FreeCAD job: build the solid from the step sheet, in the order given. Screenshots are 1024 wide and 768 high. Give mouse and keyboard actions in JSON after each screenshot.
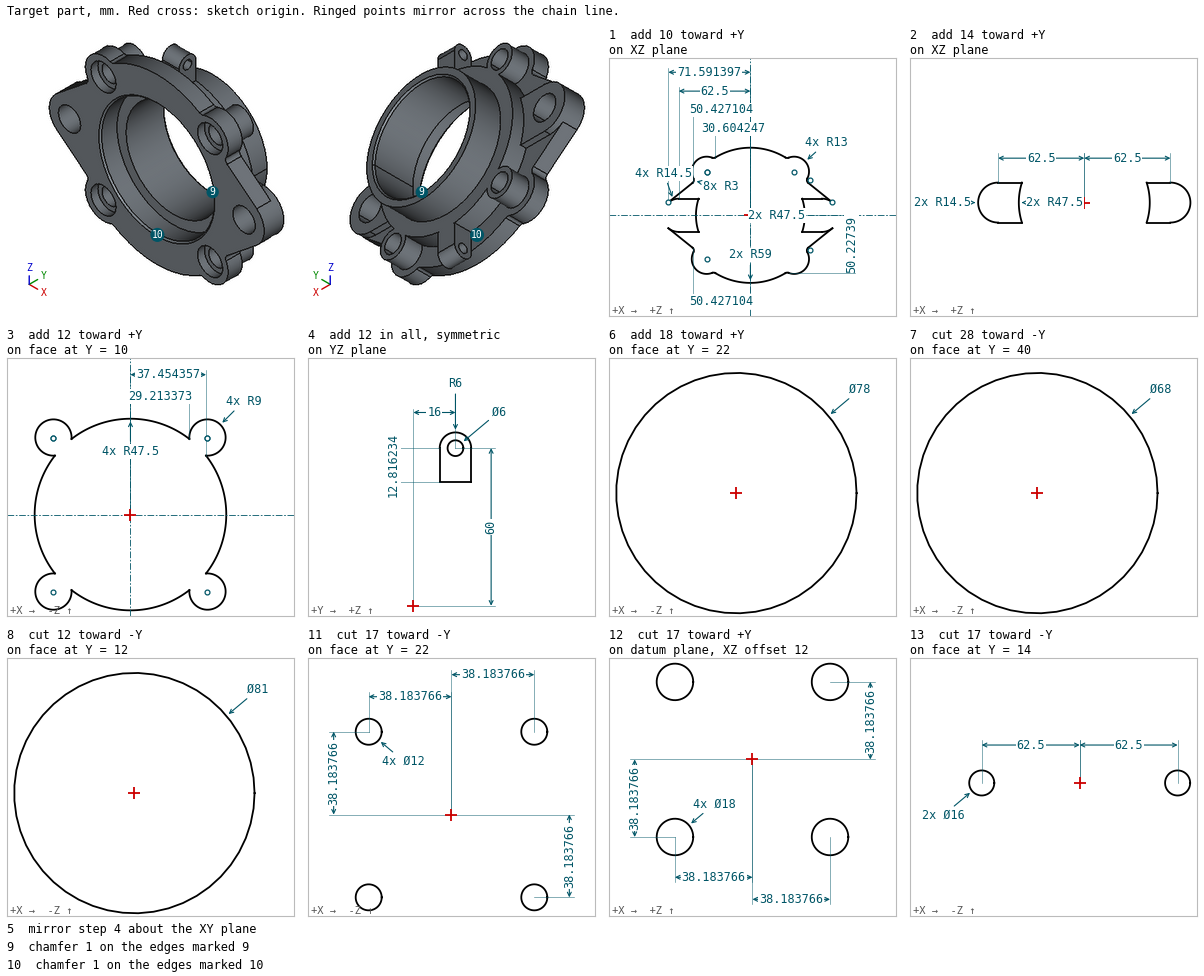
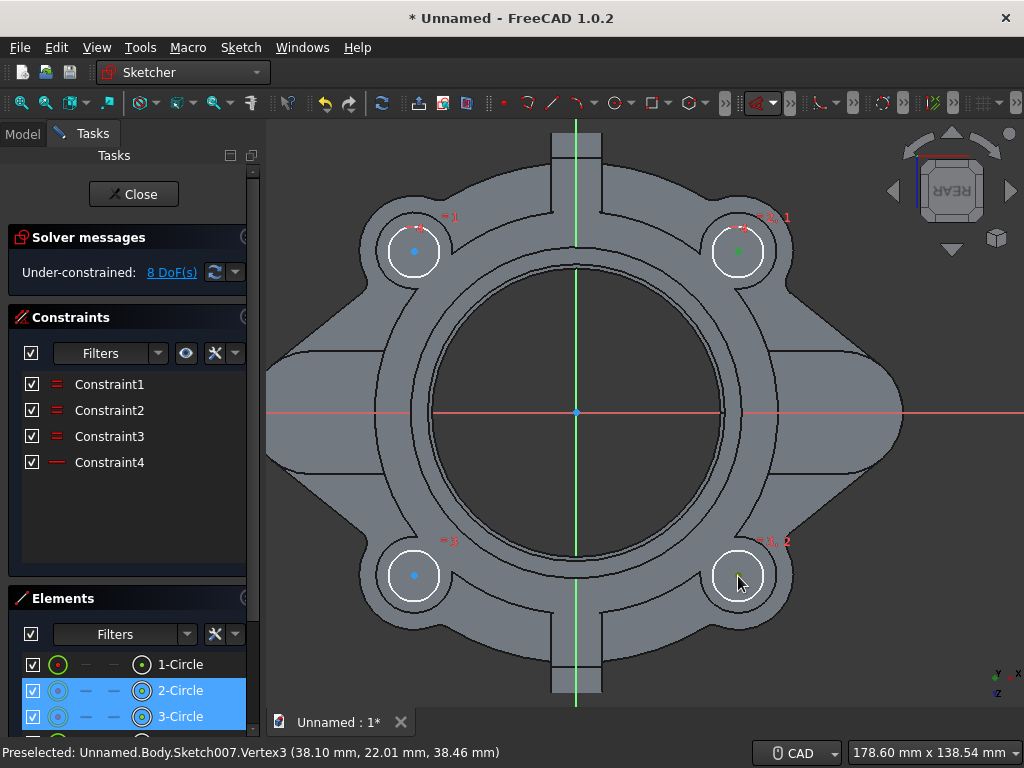
{"action": "key", "text": "v"}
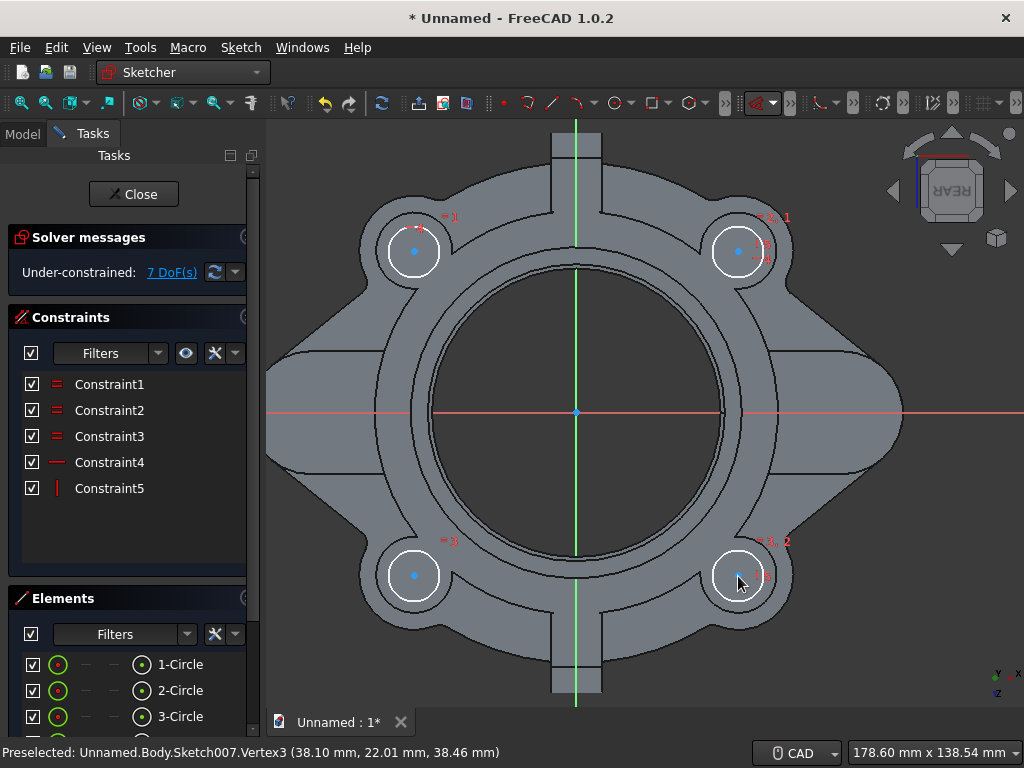
{"action": "left_click", "coordinate": [414, 252]}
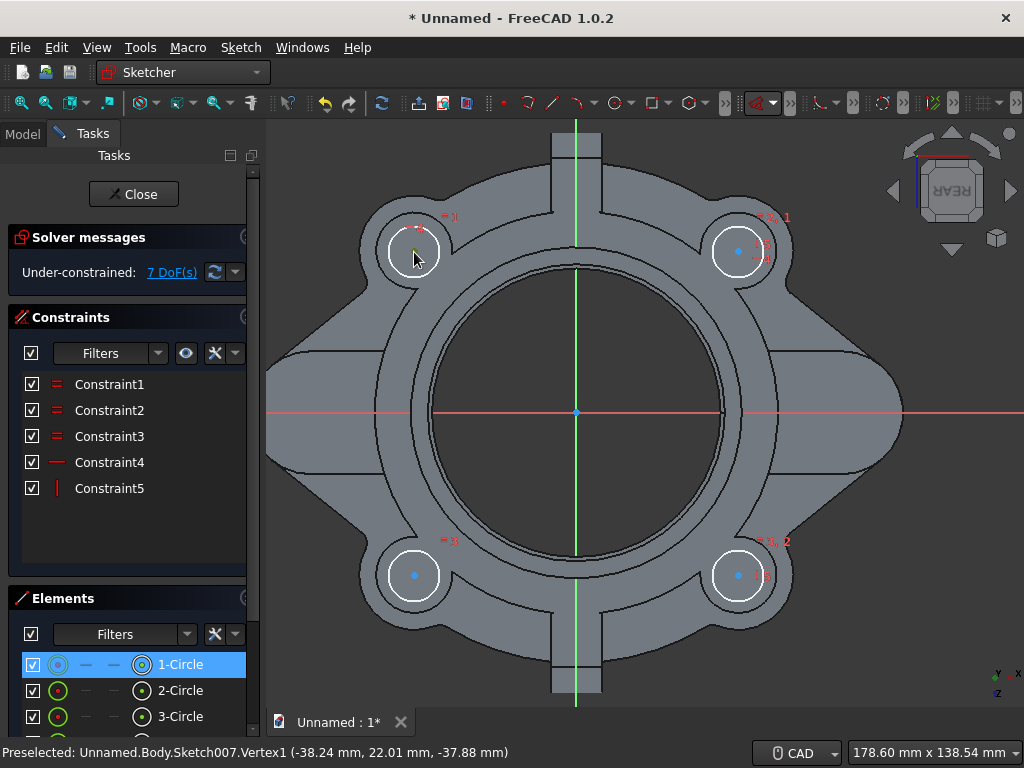
{"action": "left_click", "coordinate": [414, 576]}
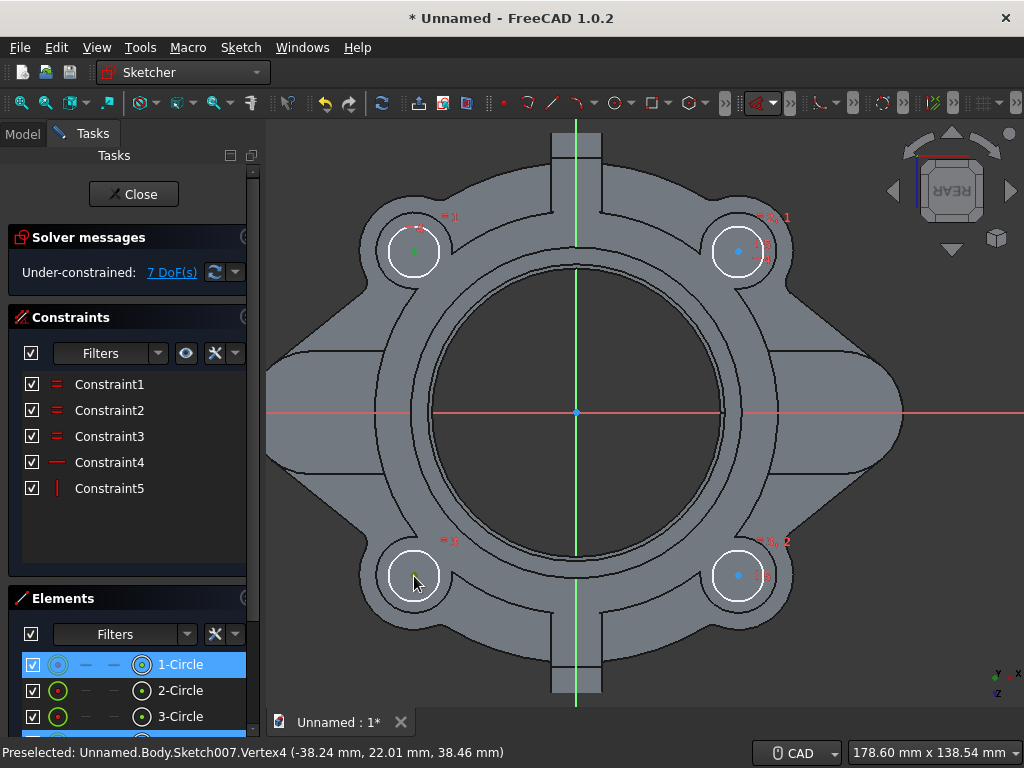
{"action": "key", "text": "v"}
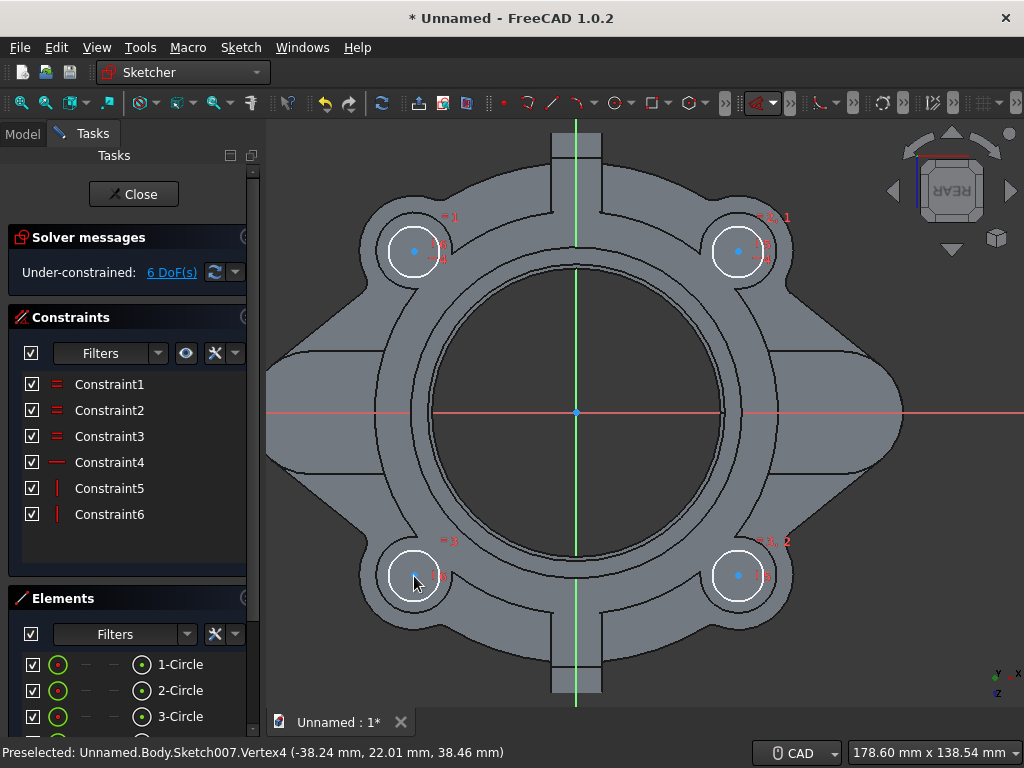
{"action": "left_click", "coordinate": [738, 576]}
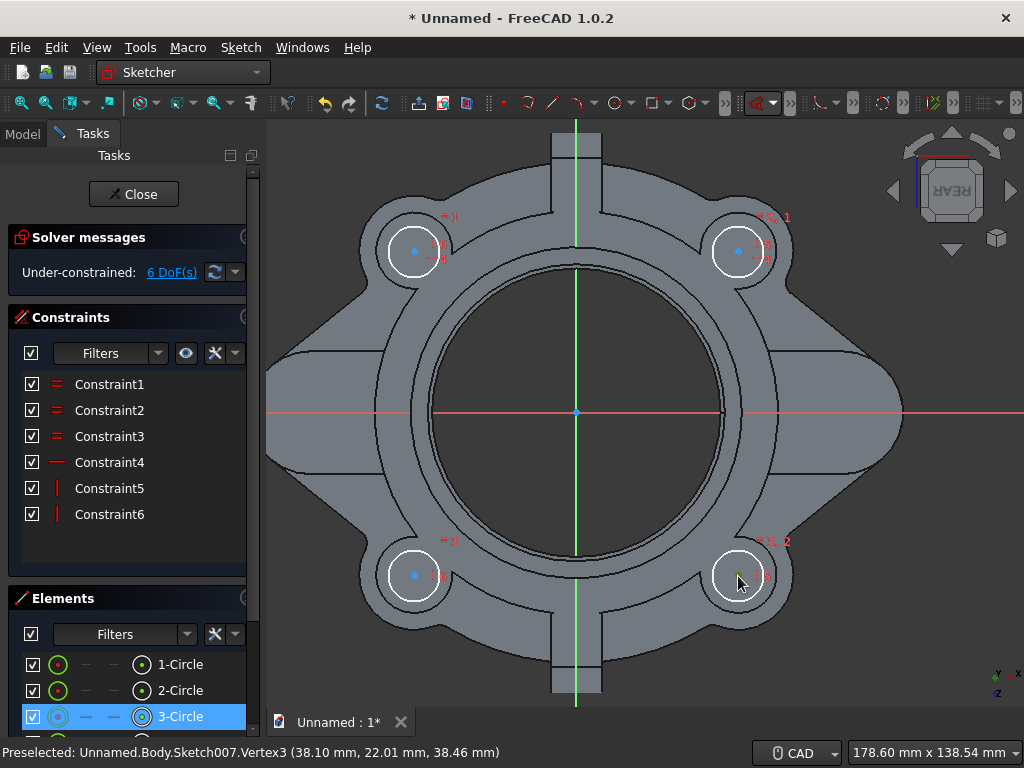
{"action": "left_click", "coordinate": [414, 576]}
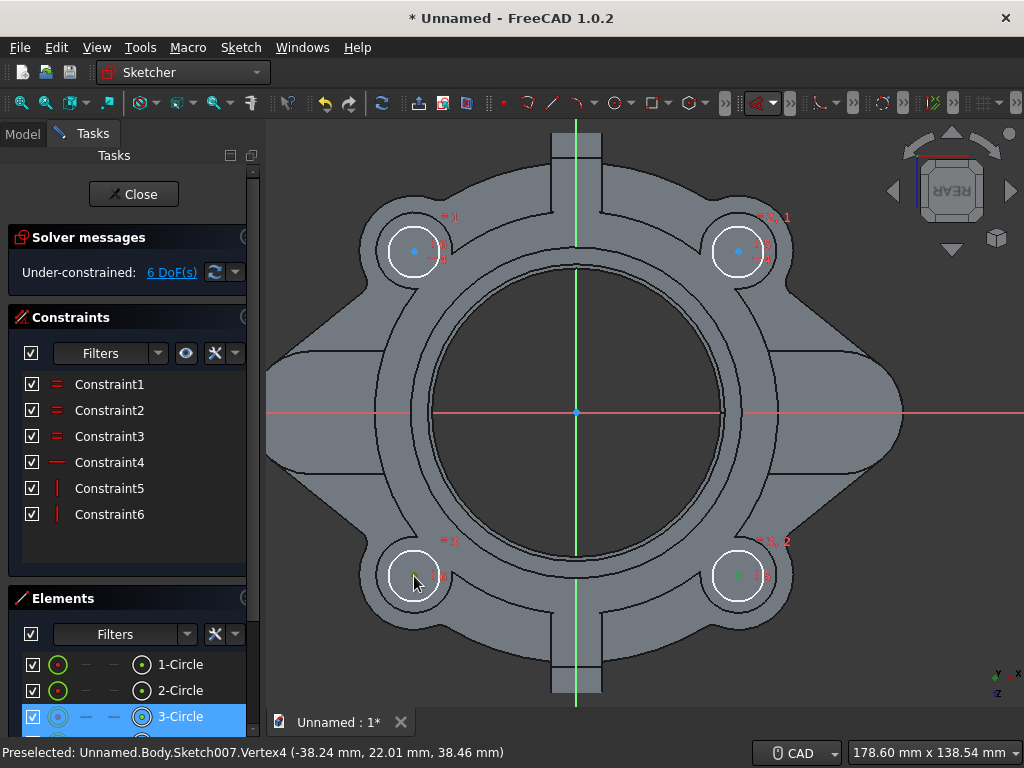
{"action": "key", "text": "h"}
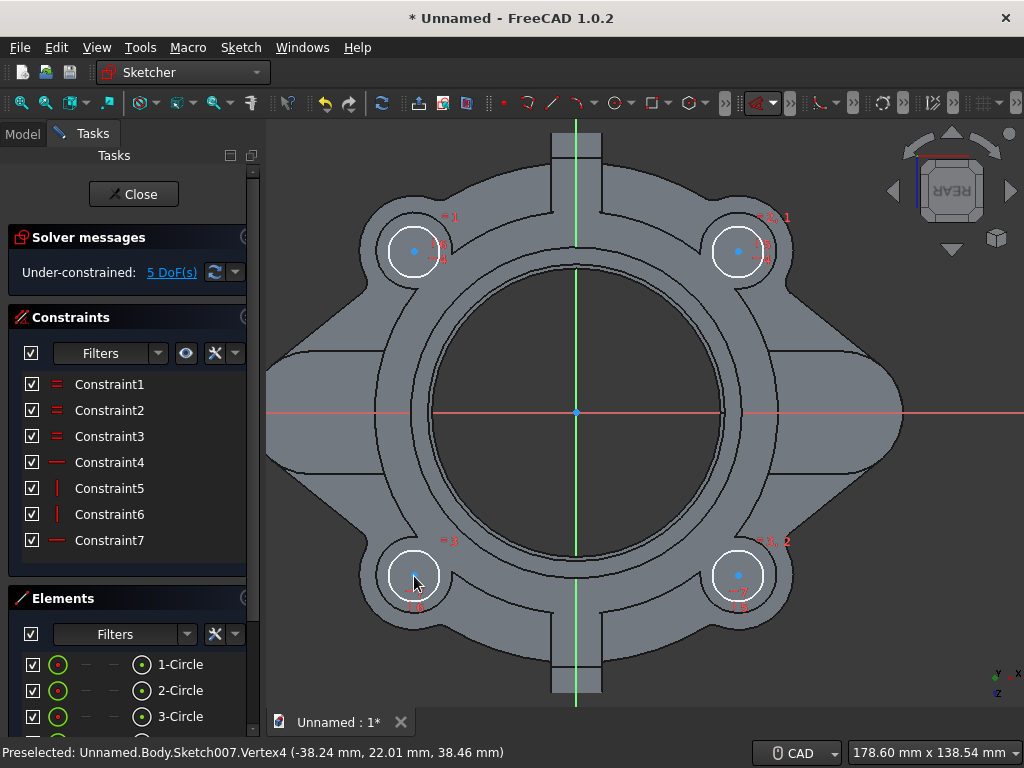
{"action": "key", "text": "d"}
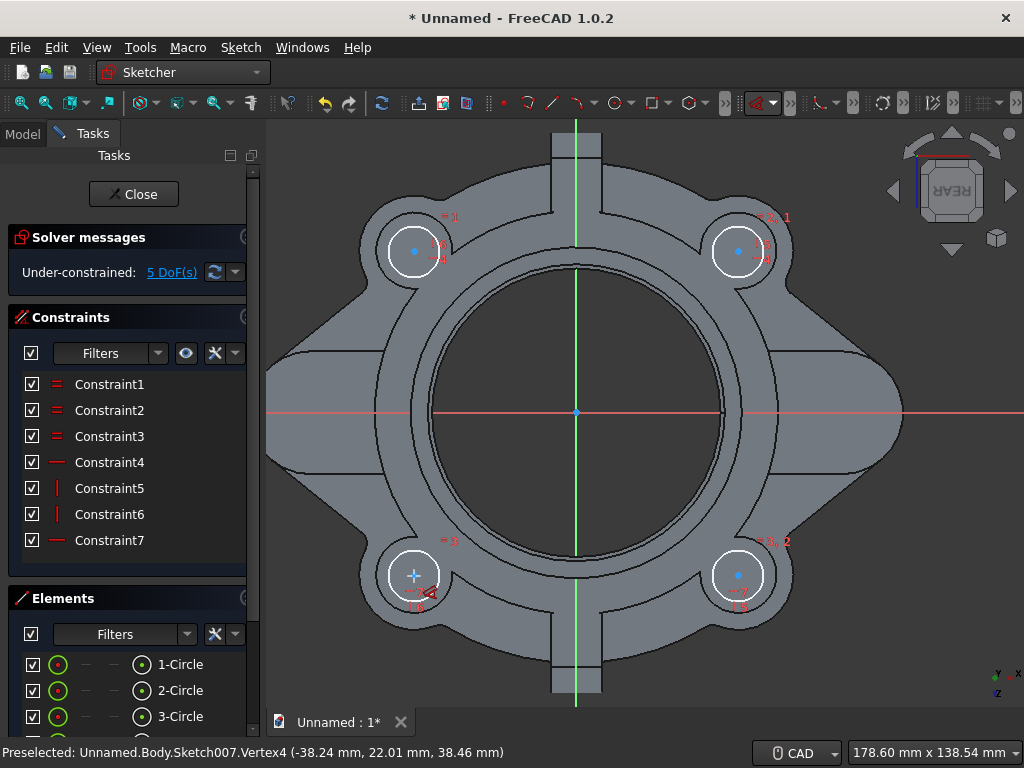
{"action": "left_click", "coordinate": [432, 234]}
{"action": "left_click", "coordinate": [455, 211]}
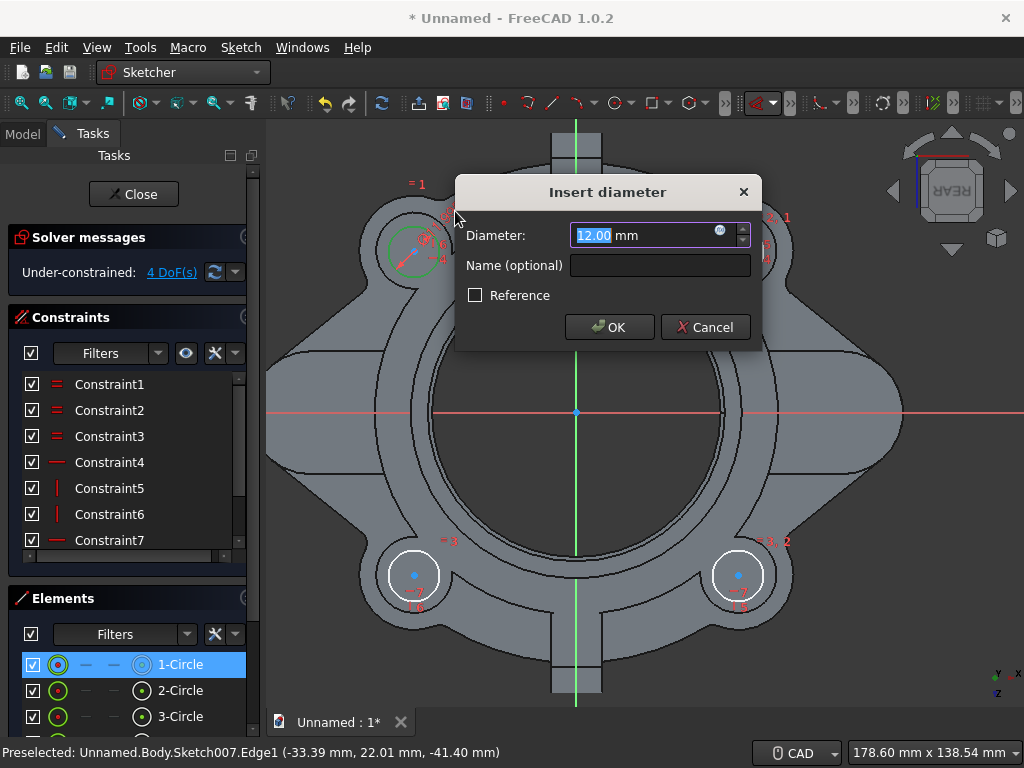
{"action": "type", "text": "12"}
{"action": "key", "text": "Return"}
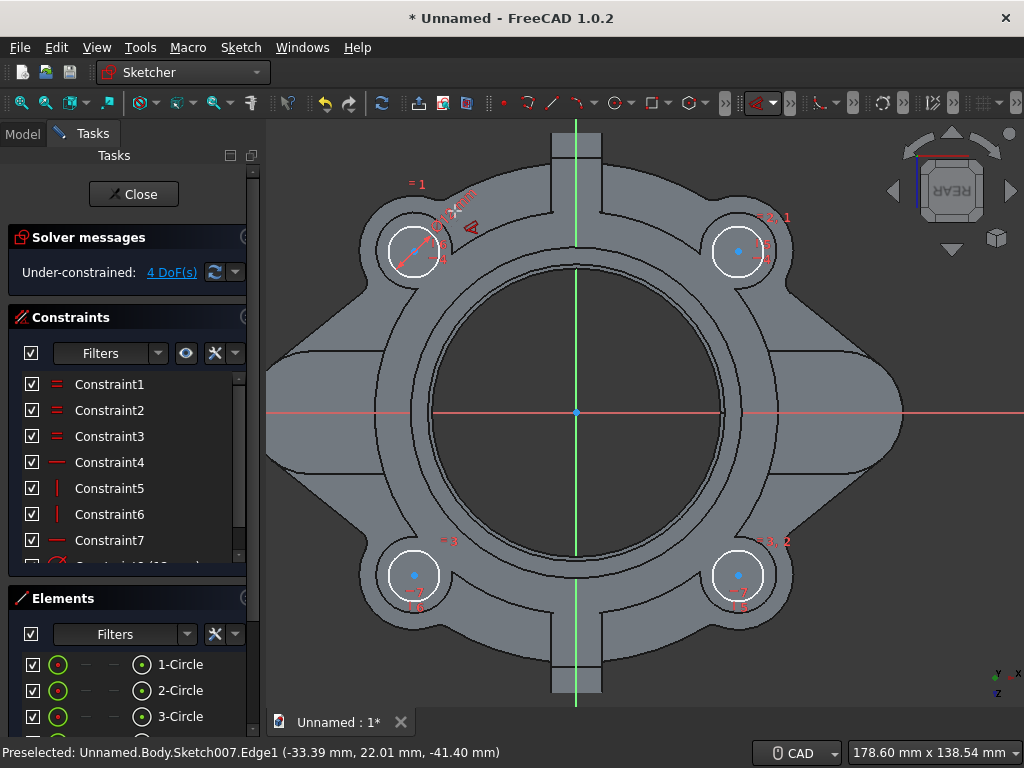
{"action": "left_click", "coordinate": [414, 252]}
{"action": "left_click", "coordinate": [532, 218]}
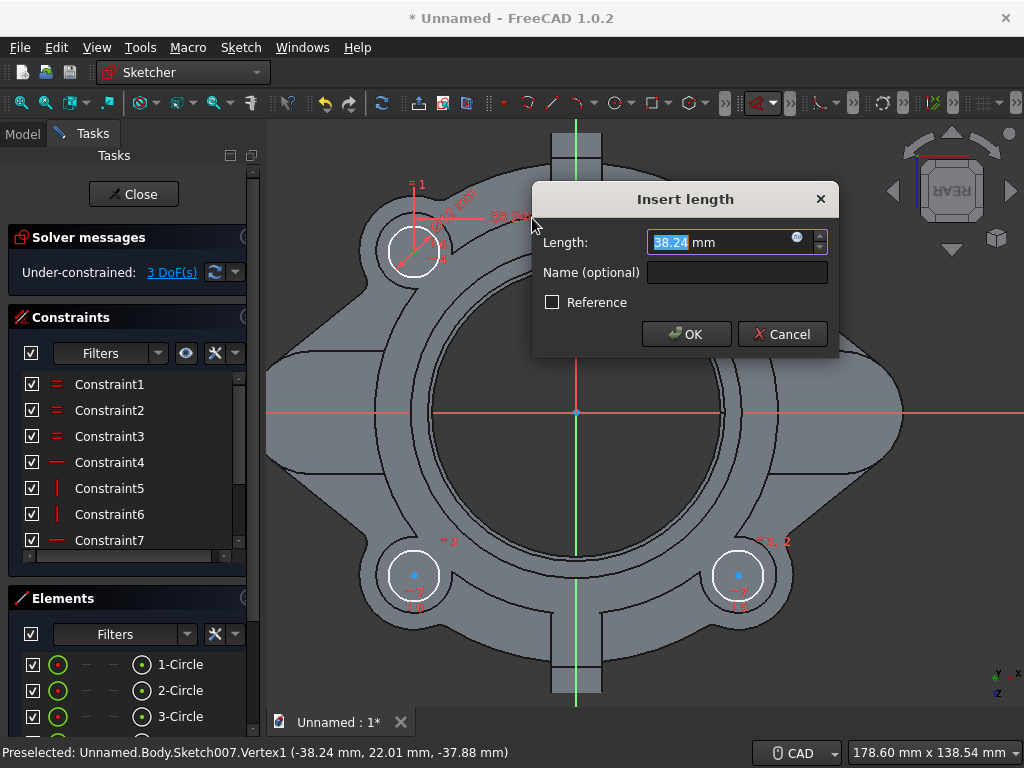
{"action": "type", "text": "38.183766"}
{"action": "key", "text": "Return"}